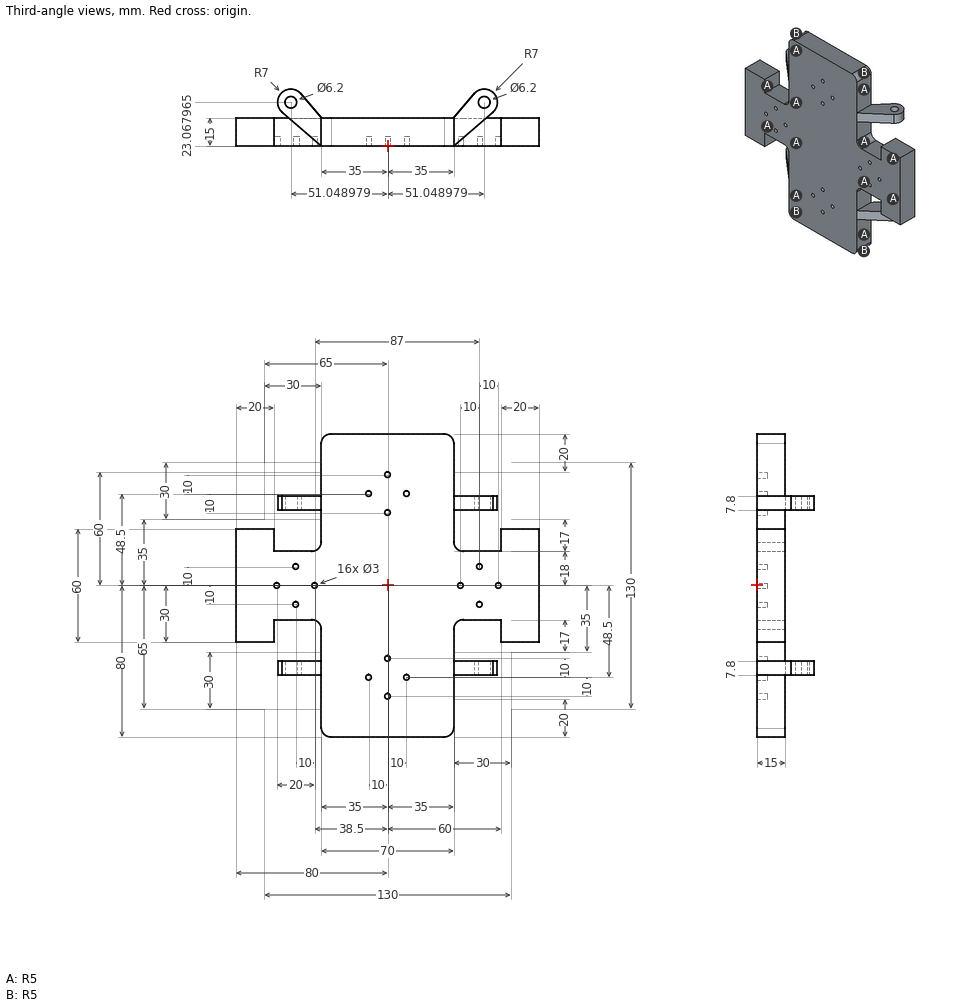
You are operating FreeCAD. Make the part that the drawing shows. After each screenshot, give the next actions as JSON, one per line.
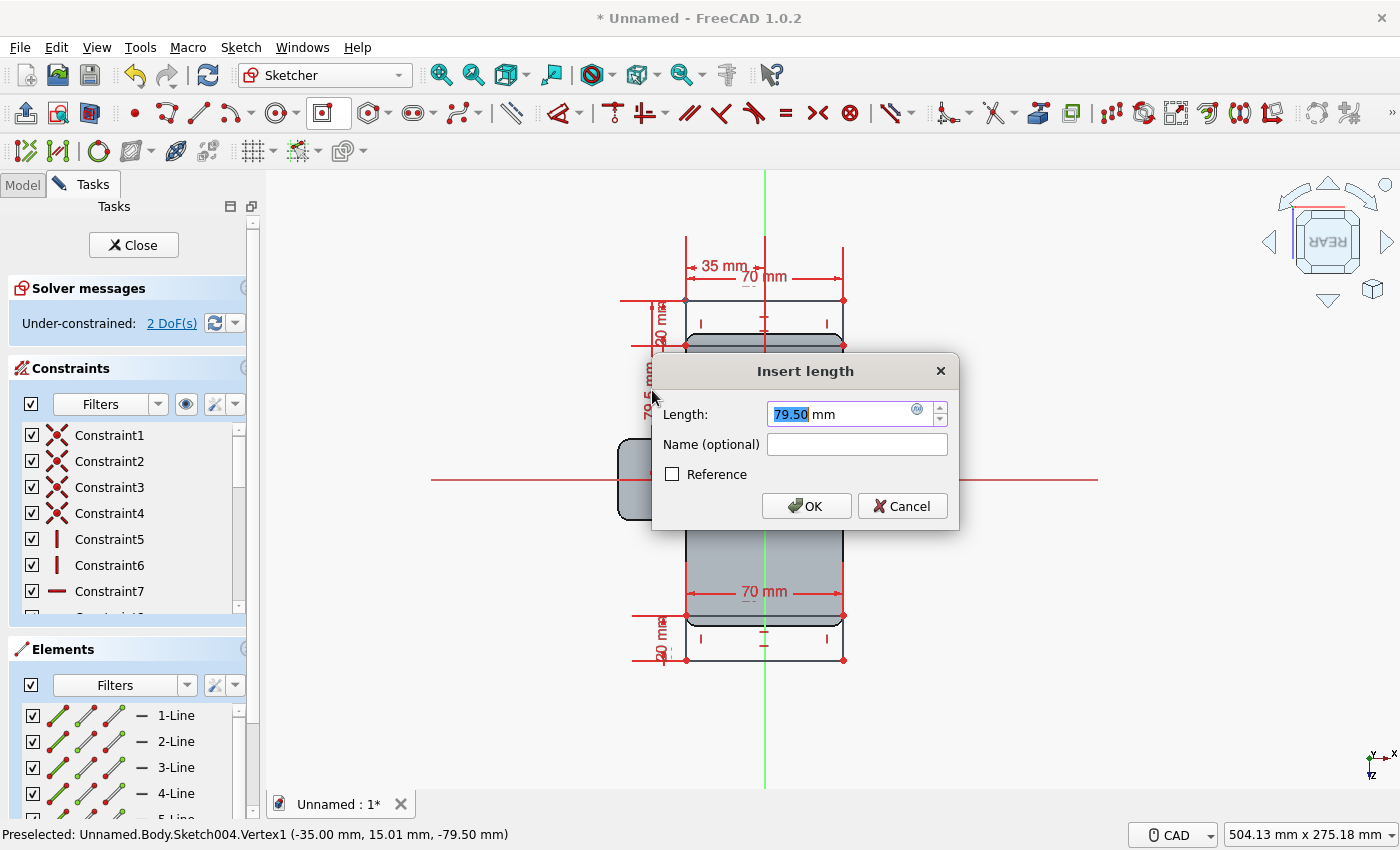
{"action": "type", "text": "80"}
{"action": "key", "text": "Return"}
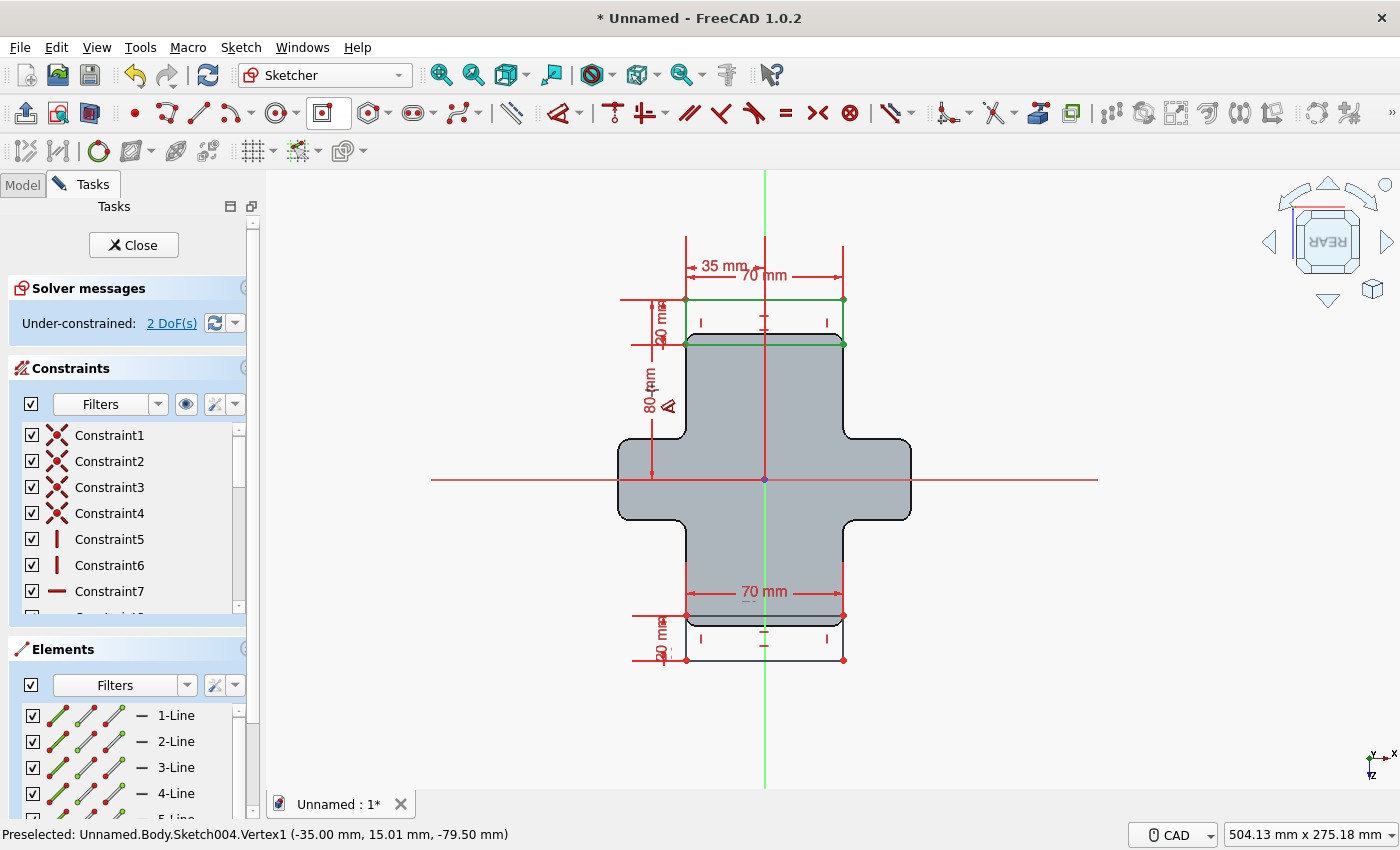
{"action": "left_click", "coordinate": [686, 616]}
{"action": "left_click", "coordinate": [725, 446]}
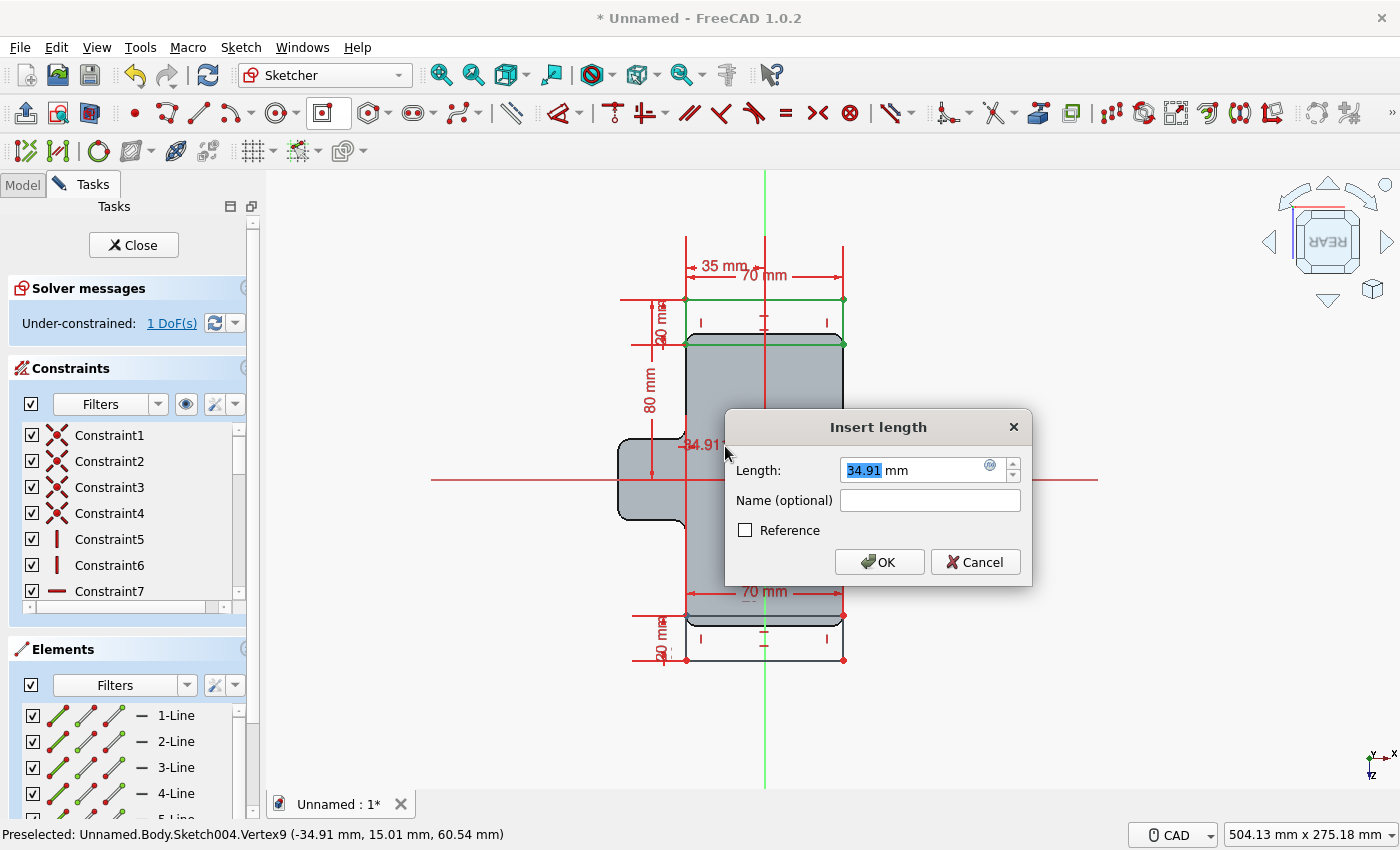
{"action": "type", "text": "35"}
{"action": "key", "text": "Return"}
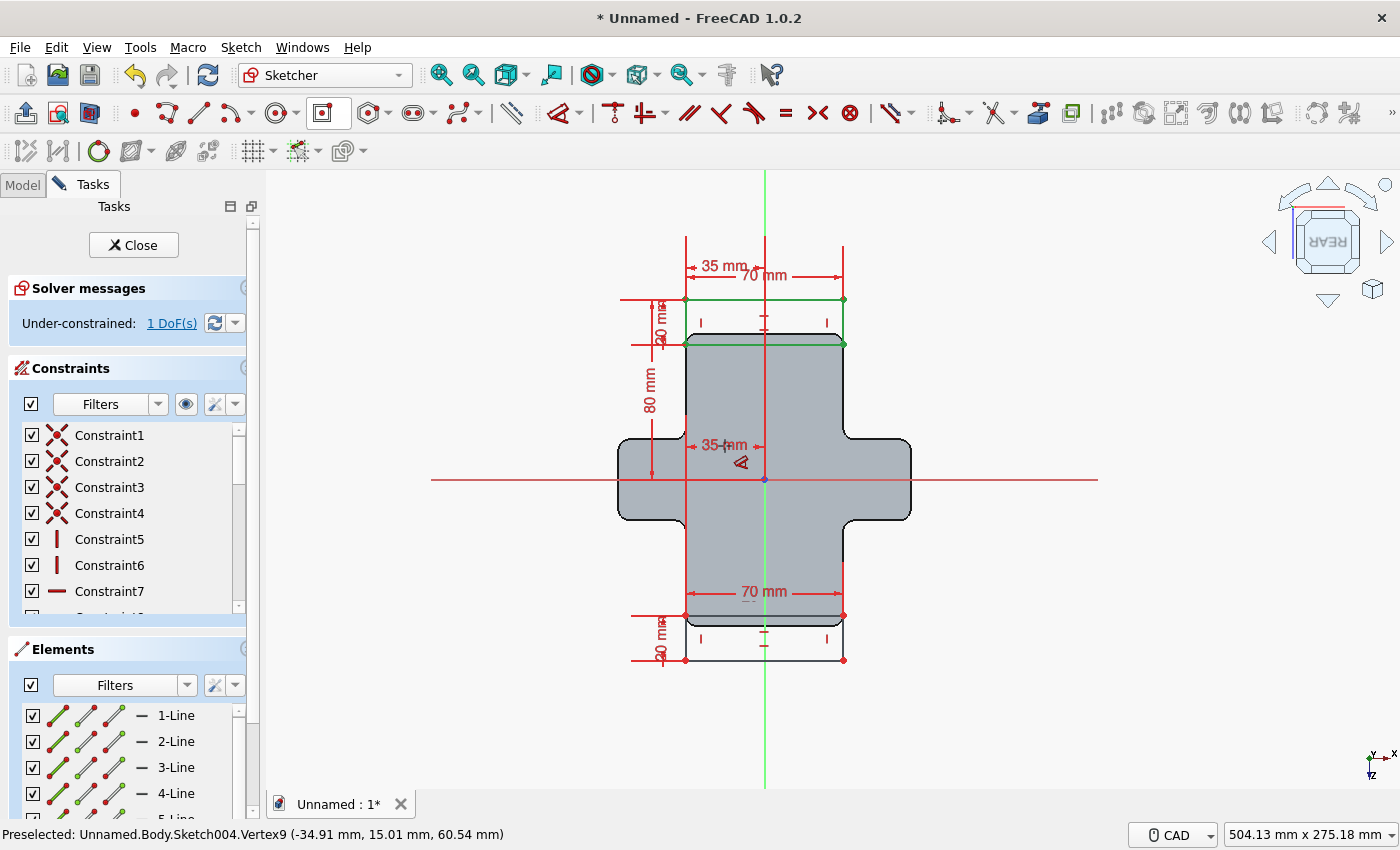
{"action": "left_click", "coordinate": [686, 616]}
{"action": "left_click", "coordinate": [652, 548]}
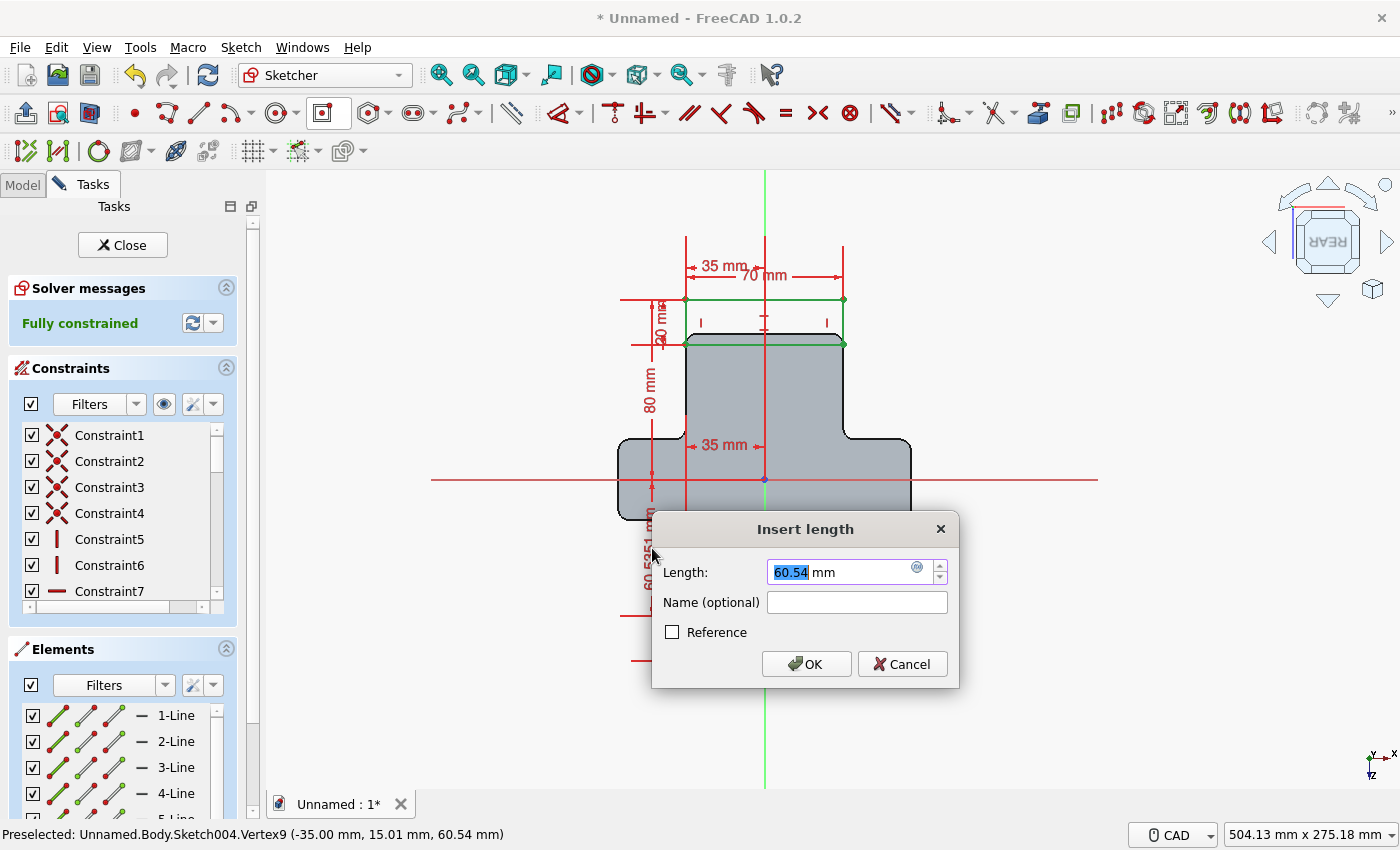
{"action": "type", "text": "60"}
{"action": "key", "text": "Return"}
{"action": "key", "text": "Escape"}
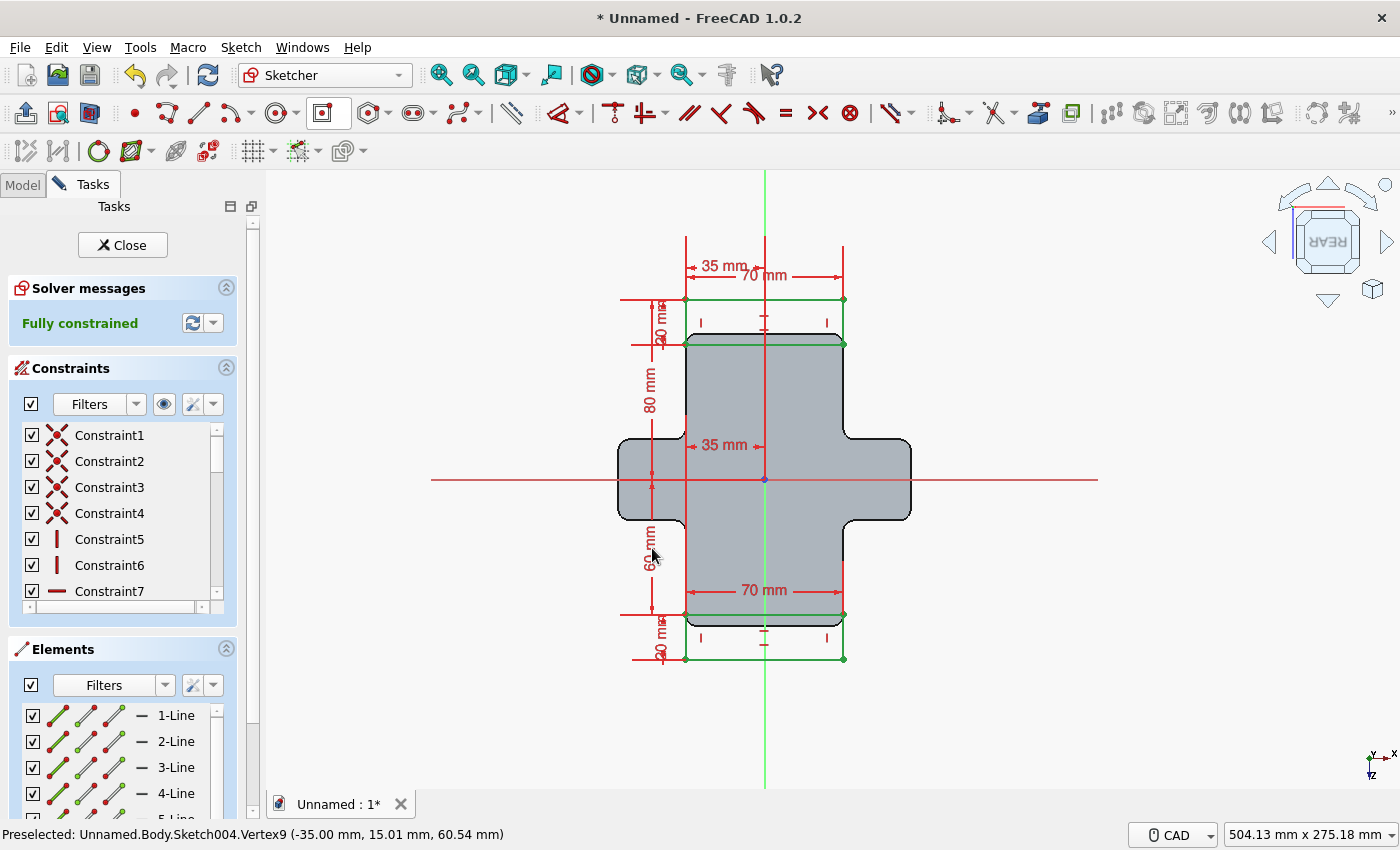
{"action": "left_click", "coordinate": [123, 245]}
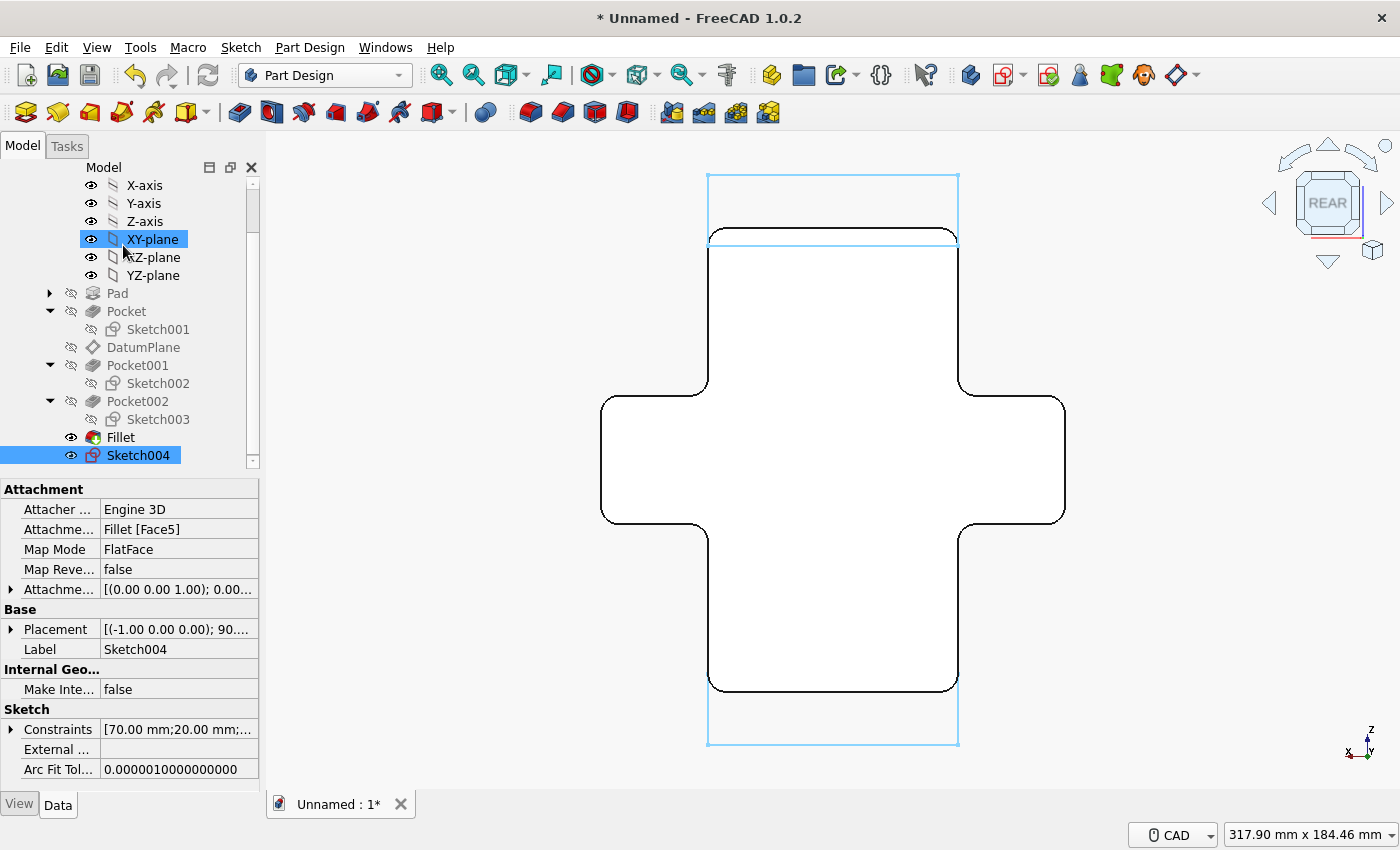
{"action": "left_click", "coordinate": [26, 112]}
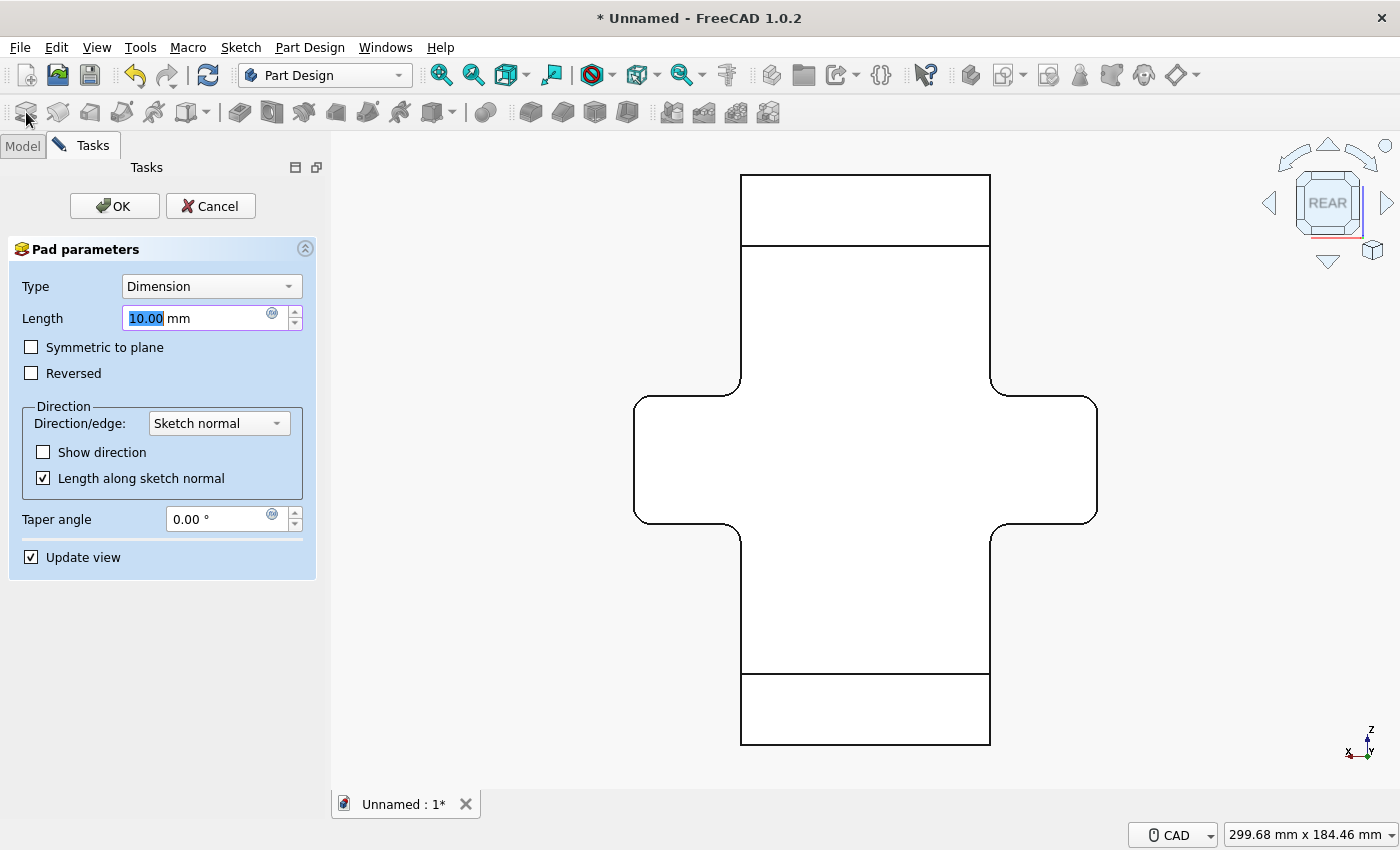
{"action": "type", "text": "15"}
{"action": "key", "text": "Tab"}